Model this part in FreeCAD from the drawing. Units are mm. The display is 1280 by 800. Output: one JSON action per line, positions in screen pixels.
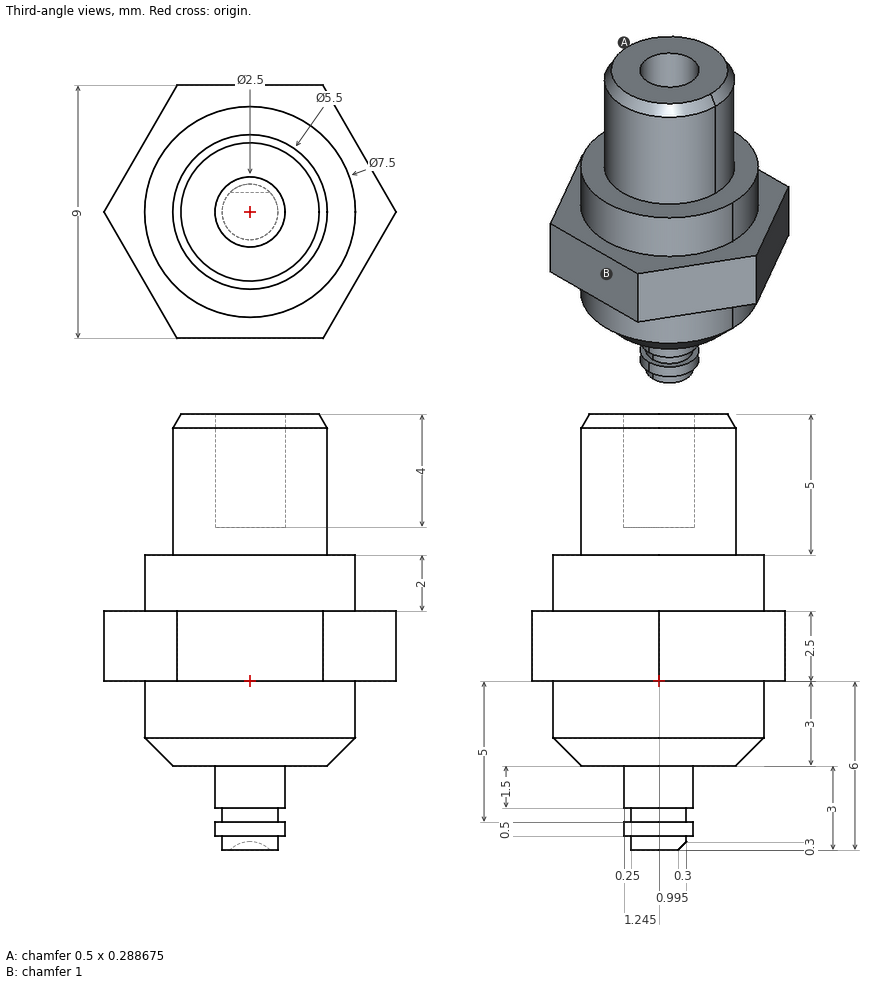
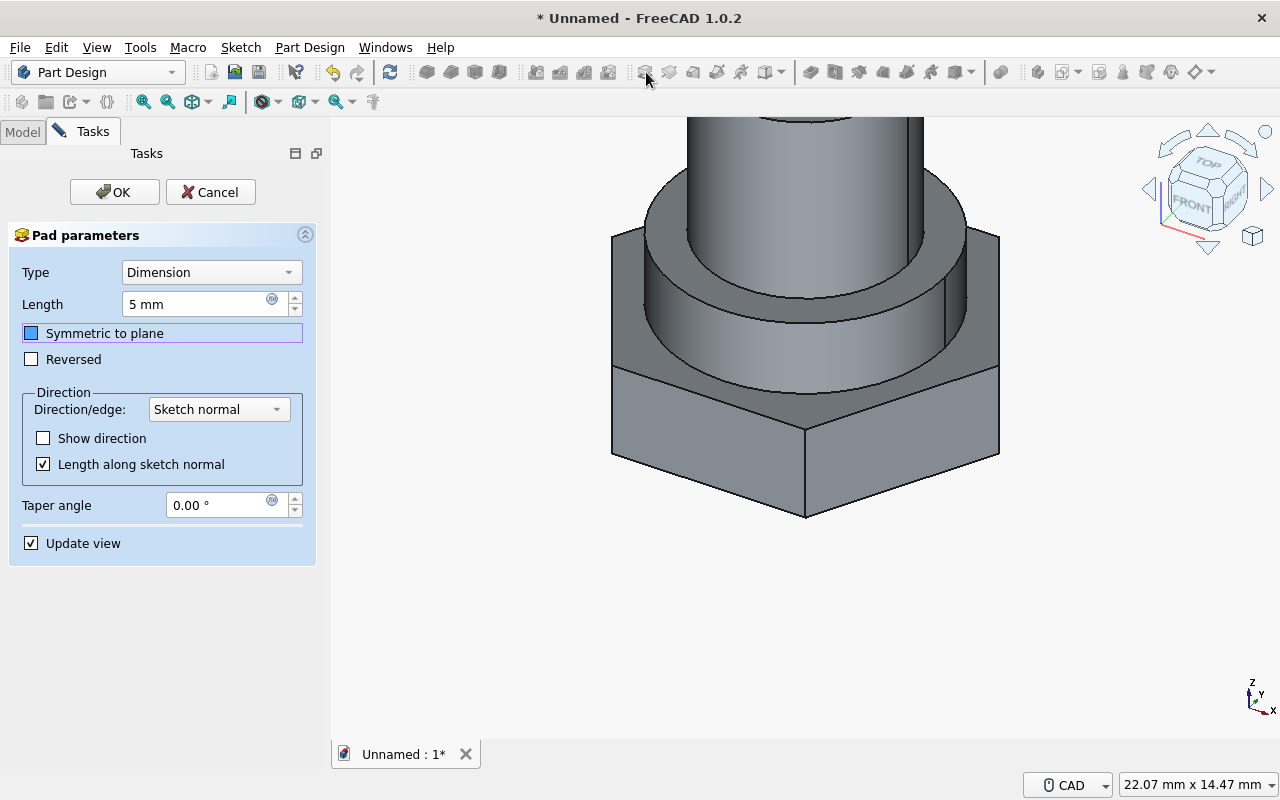
{"action": "left_click", "coordinate": [115, 192]}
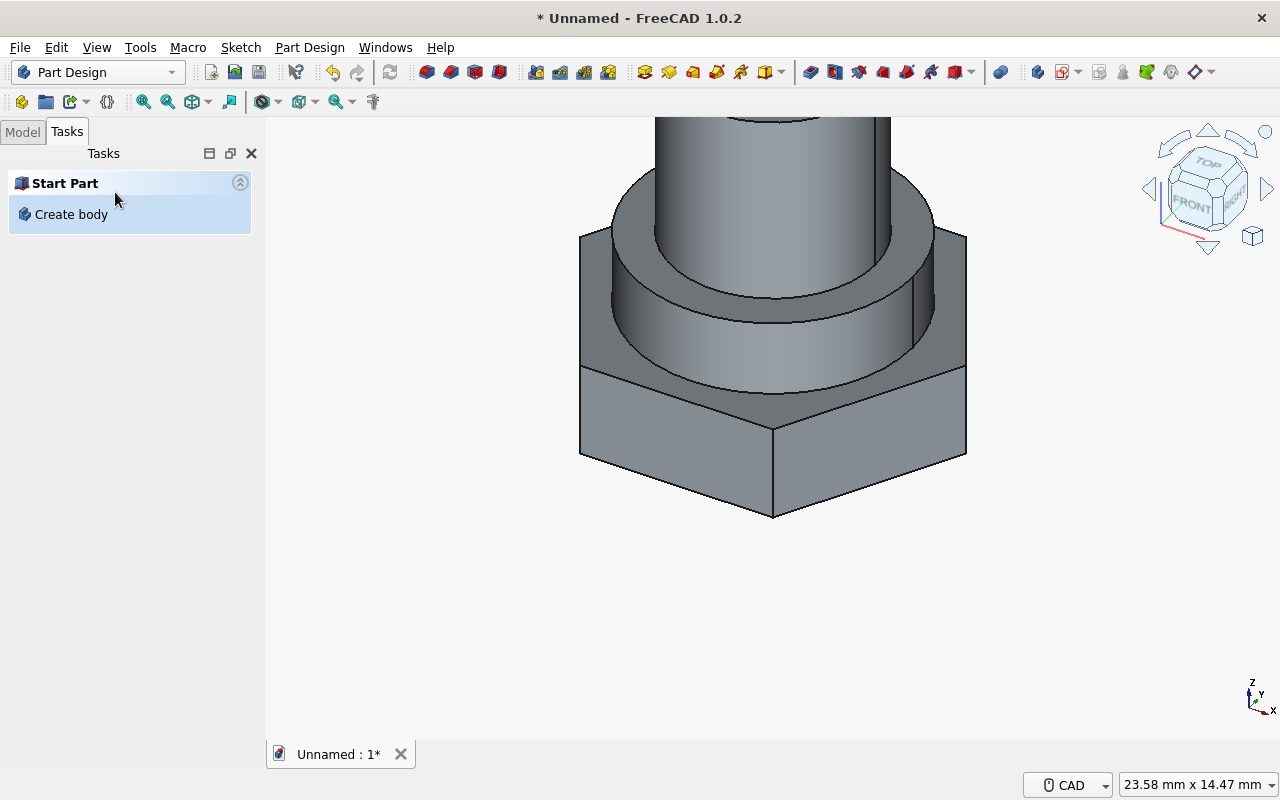
{"action": "key", "text": "v f"}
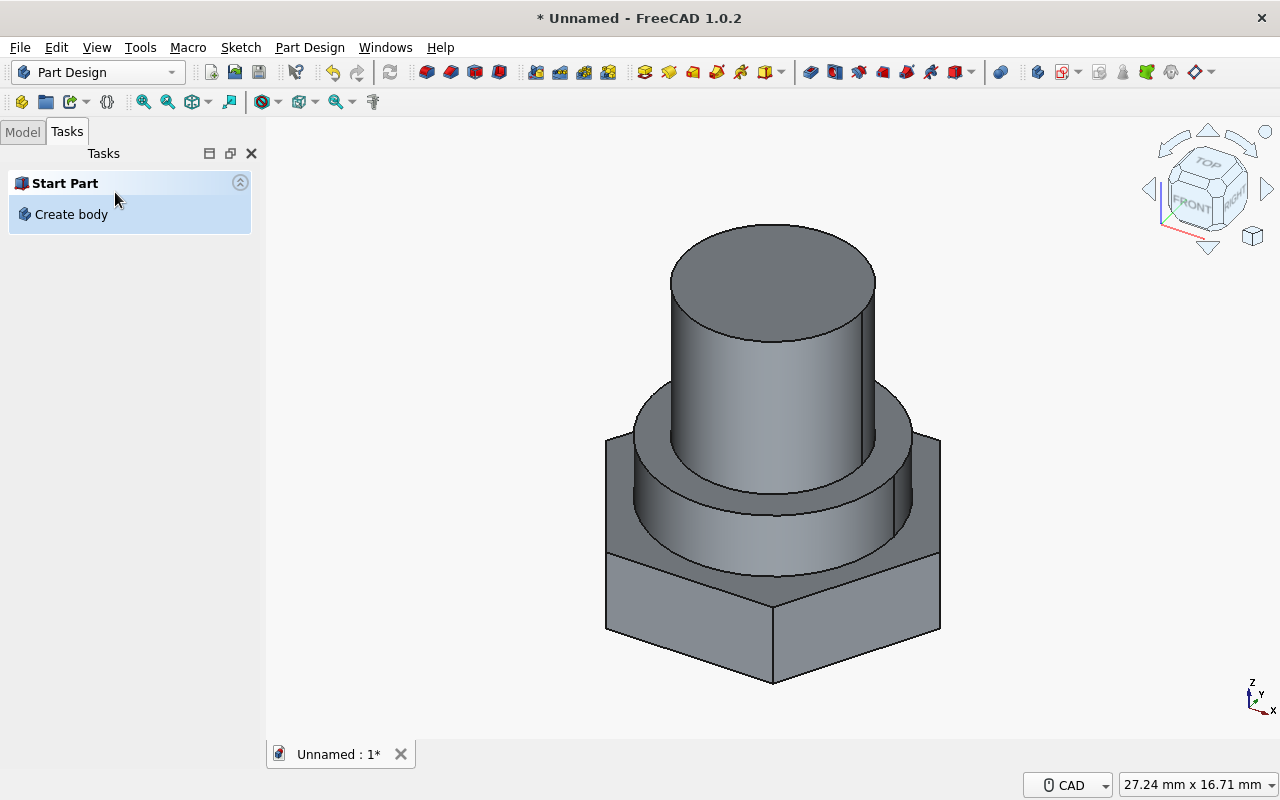
{"action": "left_click", "coordinate": [671, 288]}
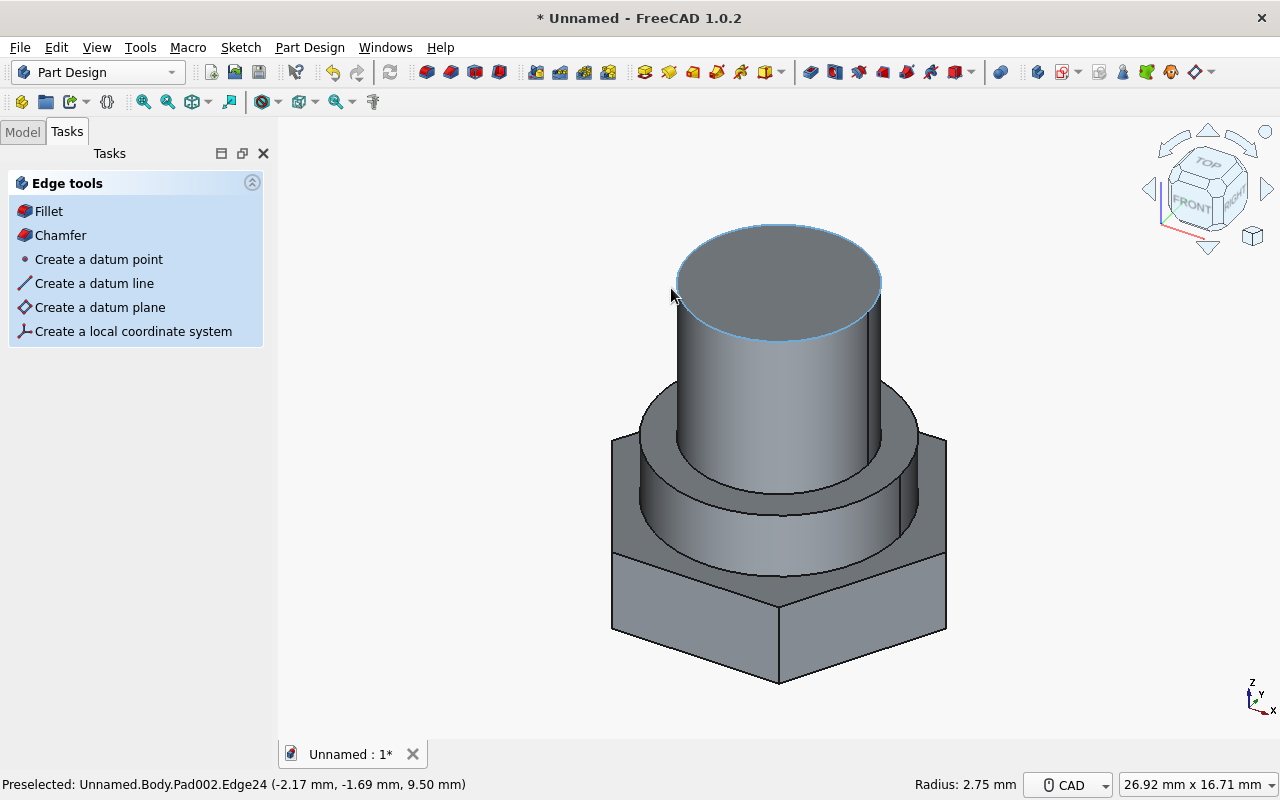
{"action": "left_click", "coordinate": [452, 72]}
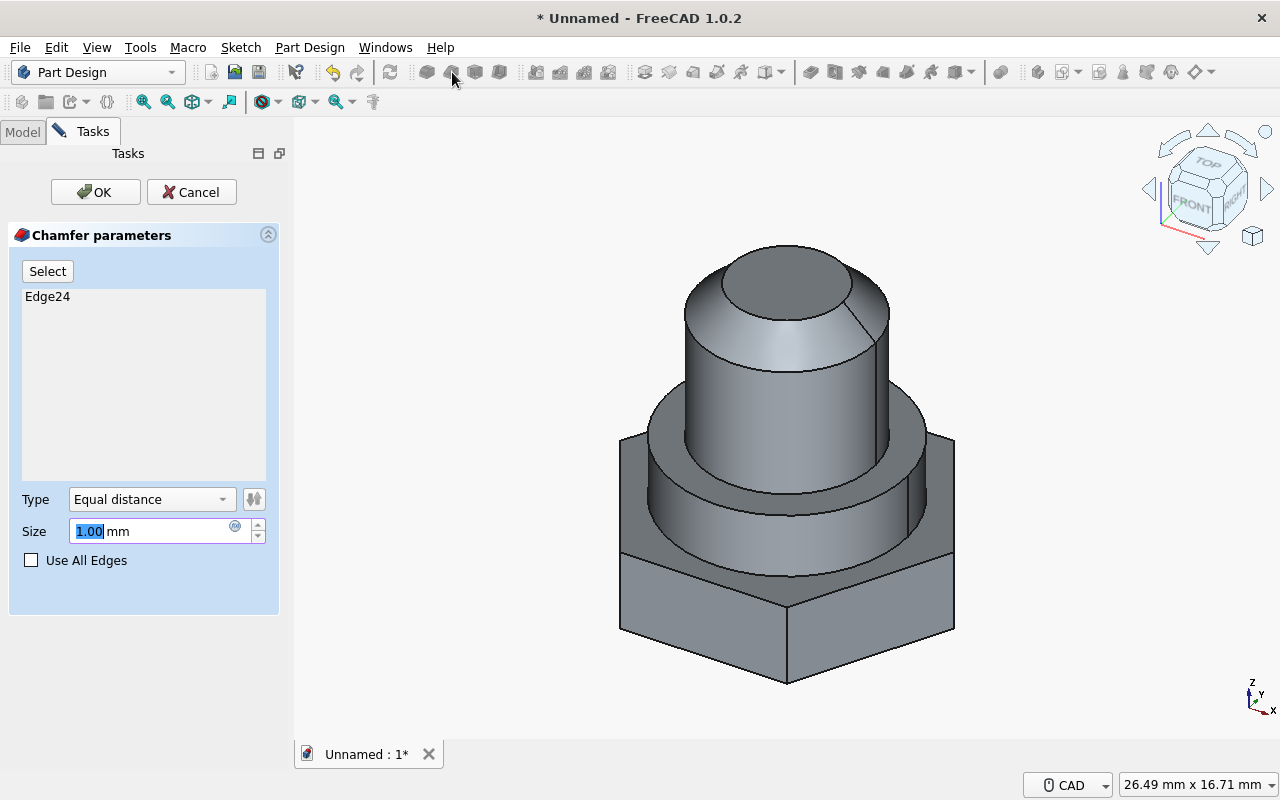
{"action": "type", "text": "0.5"}
{"action": "key", "text": "Tab"}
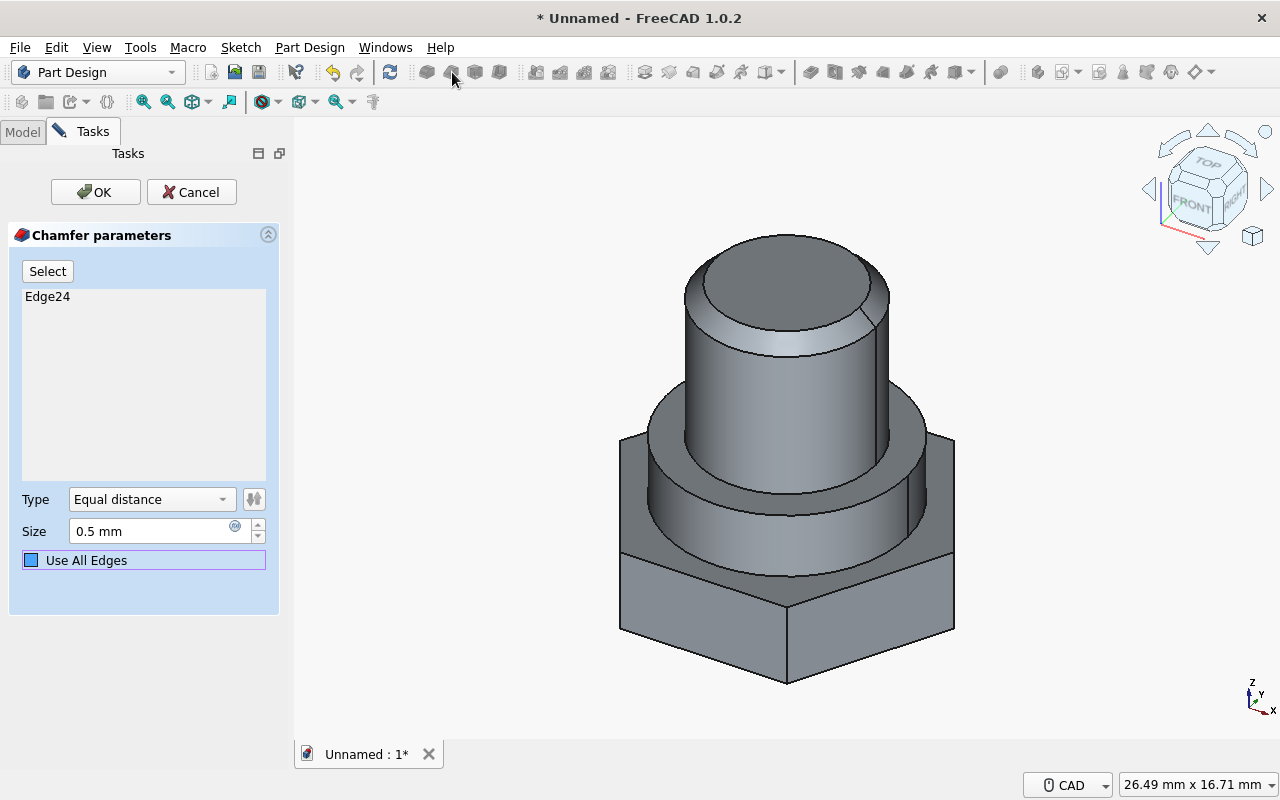
{"action": "left_click", "coordinate": [153, 500]}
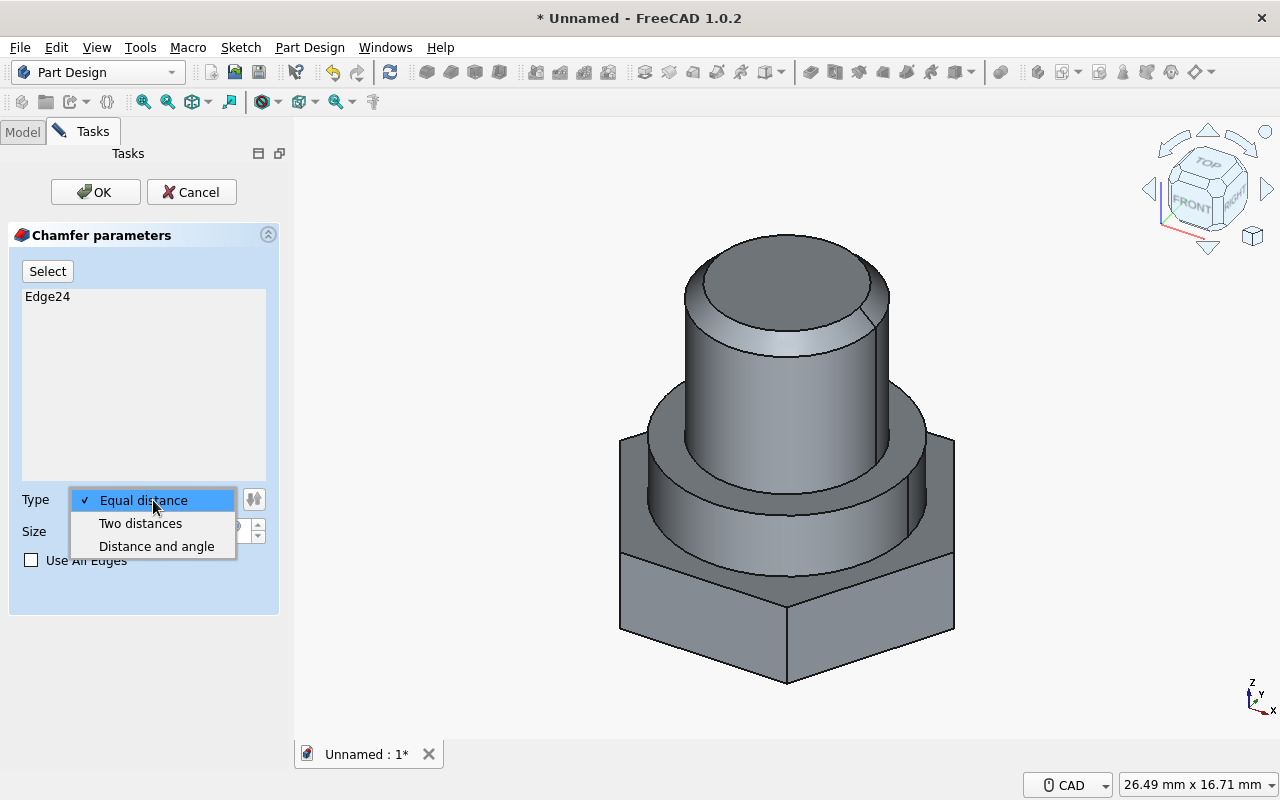
{"action": "left_click", "coordinate": [152, 524]}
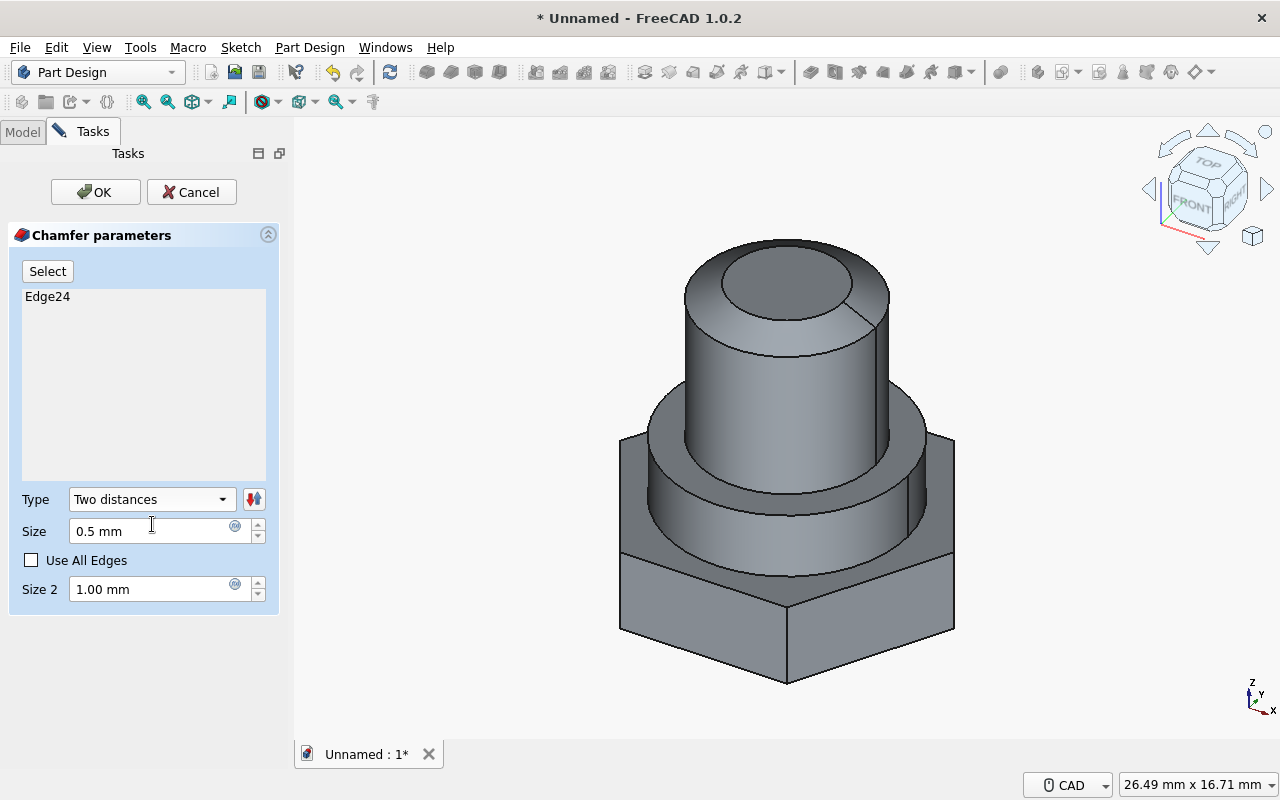
{"action": "triple_click", "coordinate": [160, 589]}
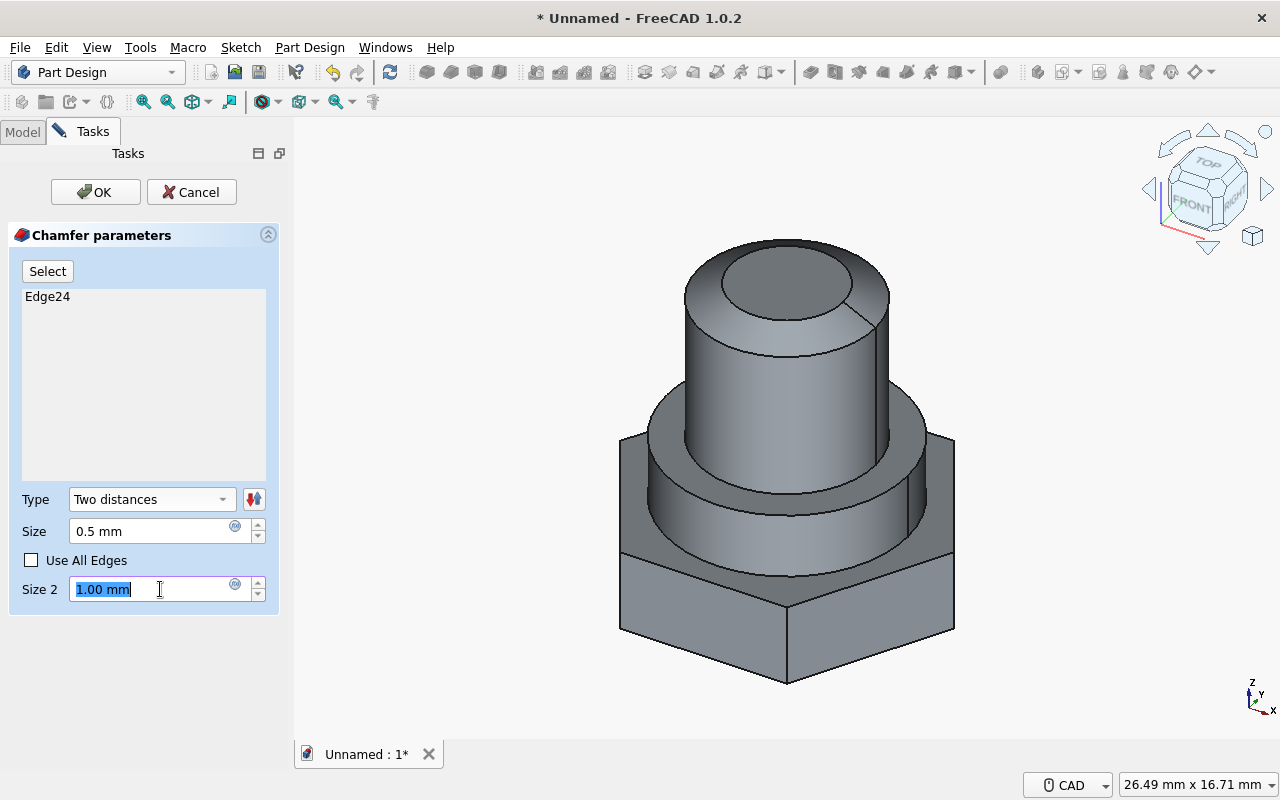
{"action": "type", "text": "0.288675"}
{"action": "key", "text": "Tab"}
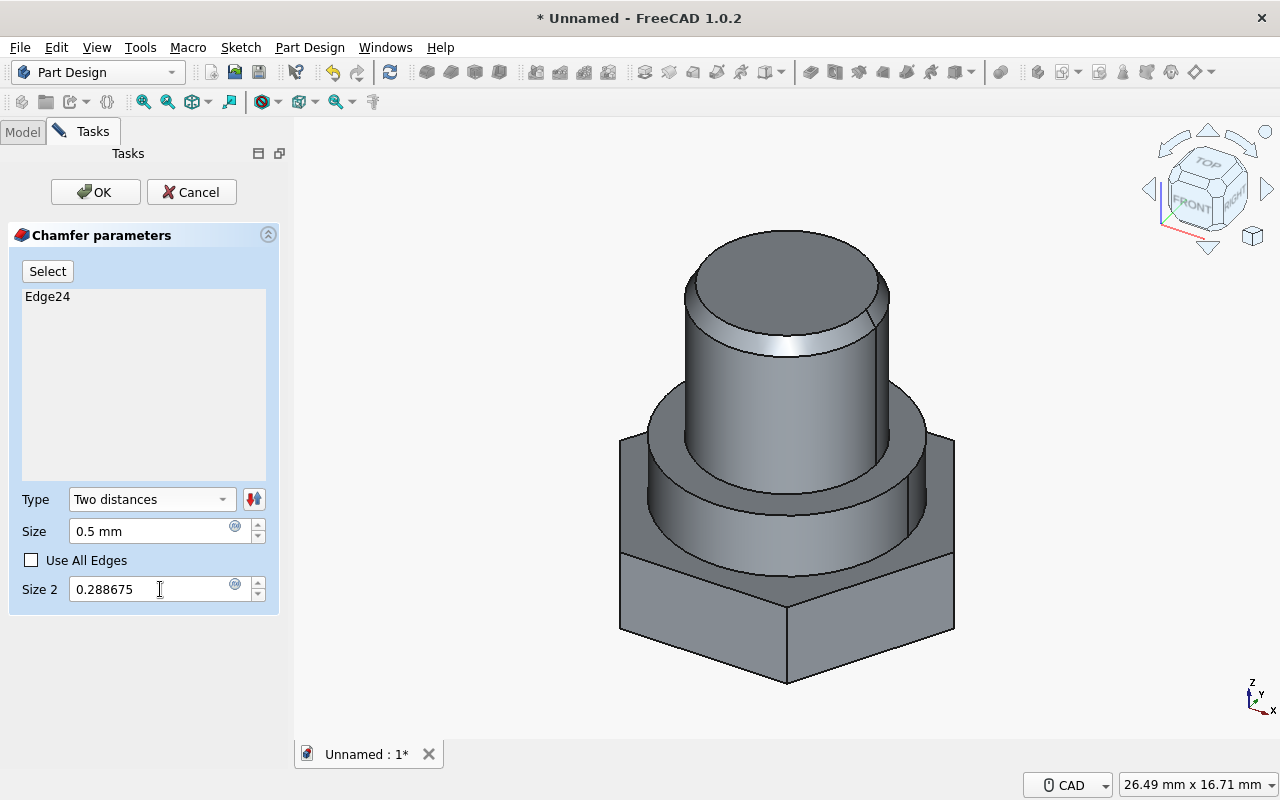
{"action": "left_click", "coordinate": [96, 192]}